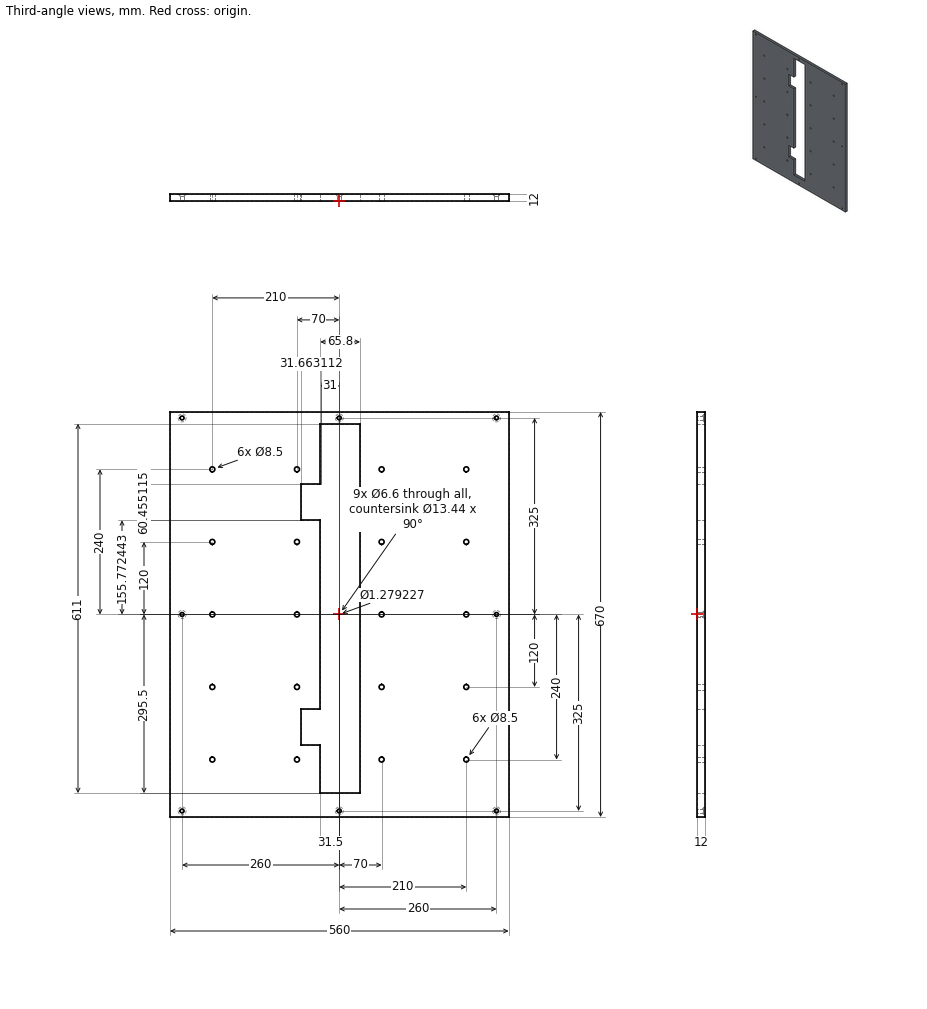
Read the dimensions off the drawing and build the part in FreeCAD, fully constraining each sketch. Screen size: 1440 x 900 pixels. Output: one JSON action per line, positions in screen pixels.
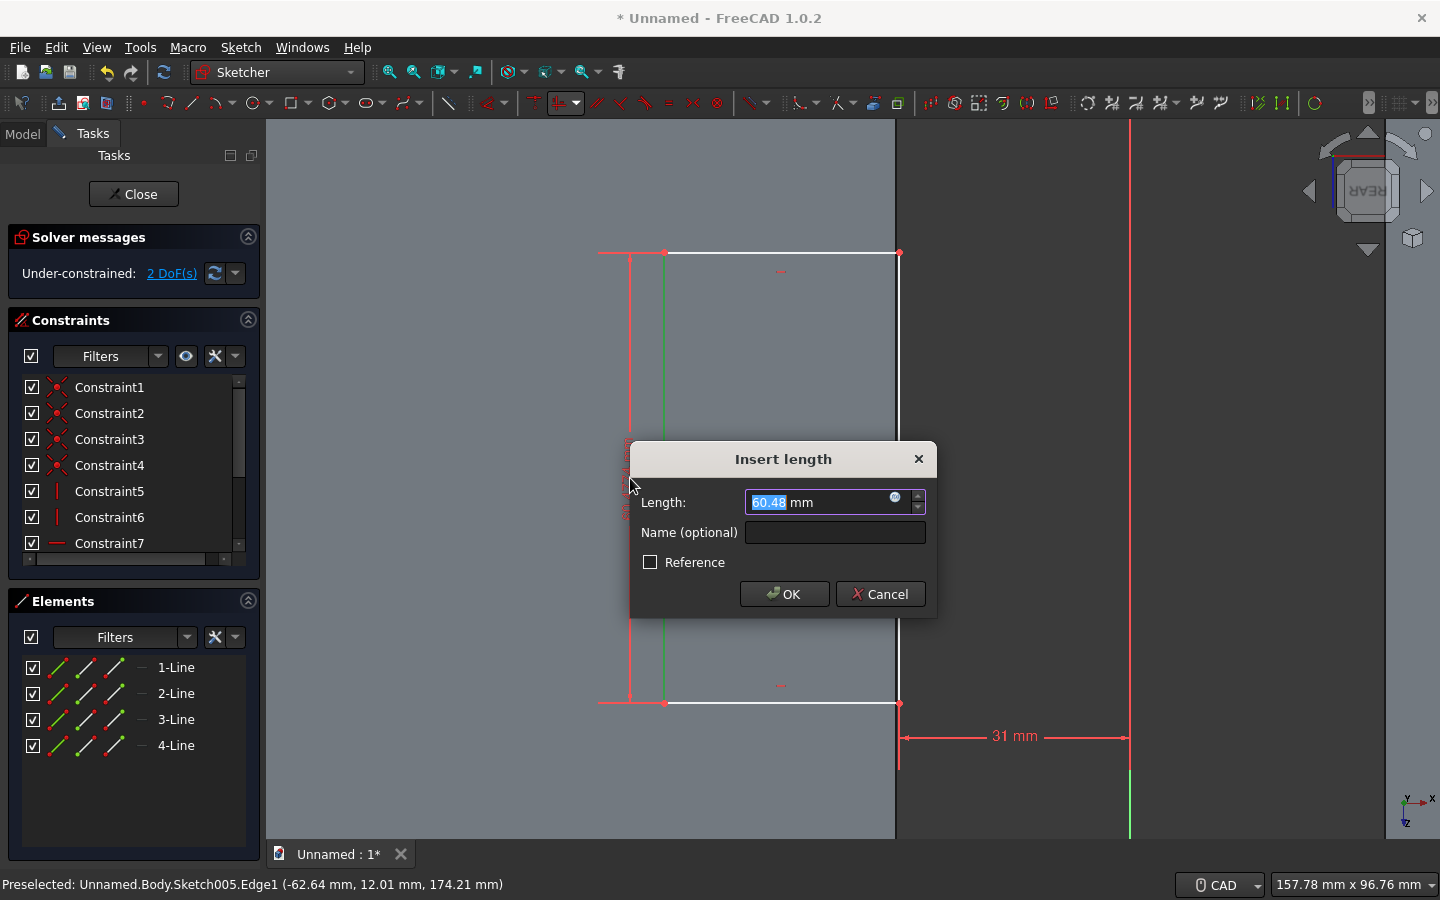
{"action": "type", "text": "60.455115"}
{"action": "key", "text": "Return"}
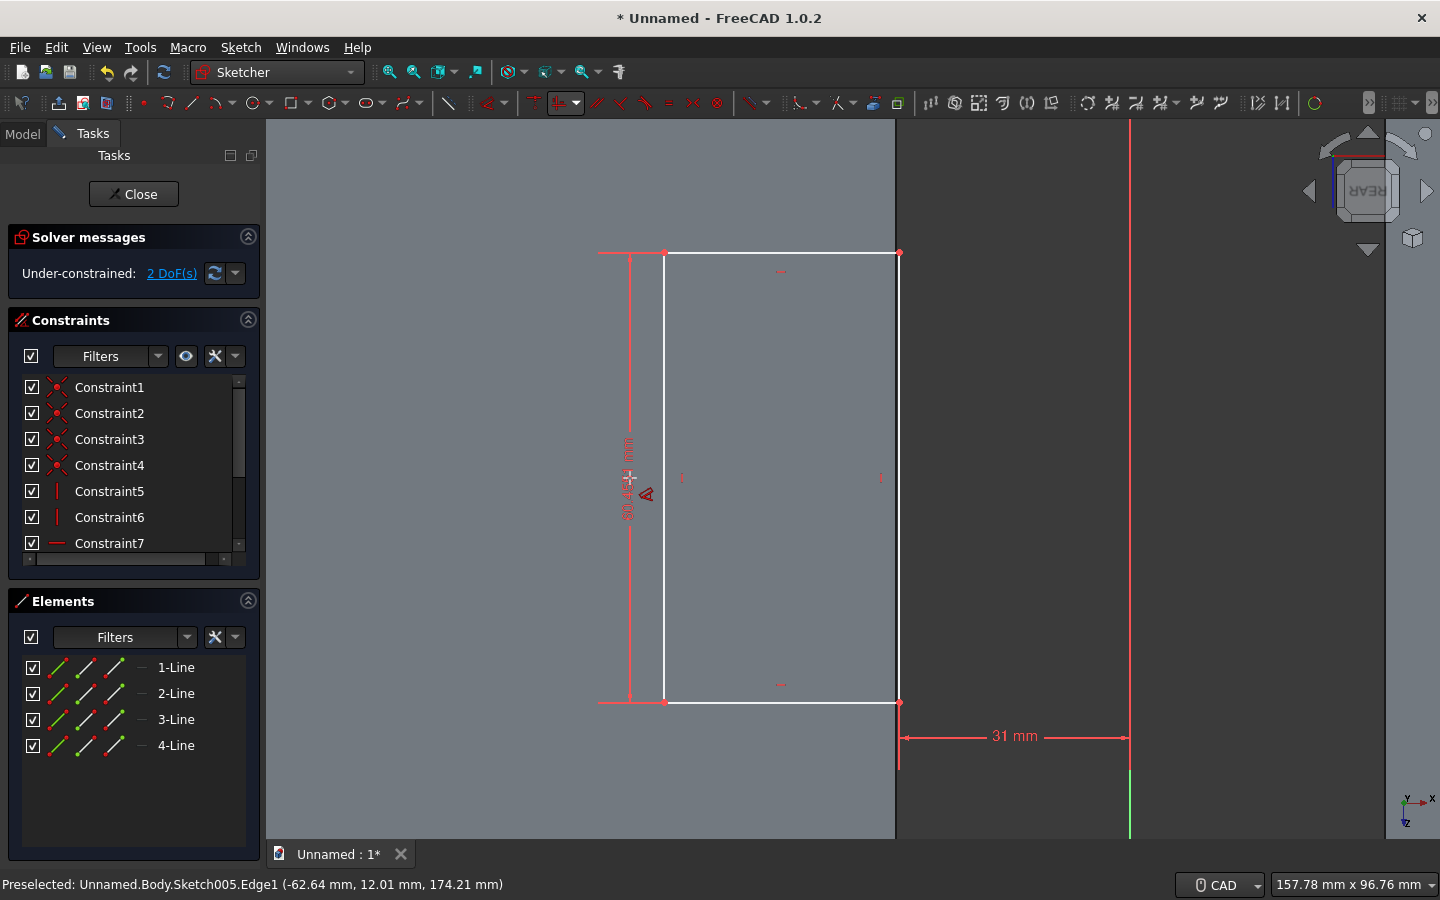
{"action": "left_click", "coordinate": [735, 703]}
{"action": "left_click", "coordinate": [782, 737]}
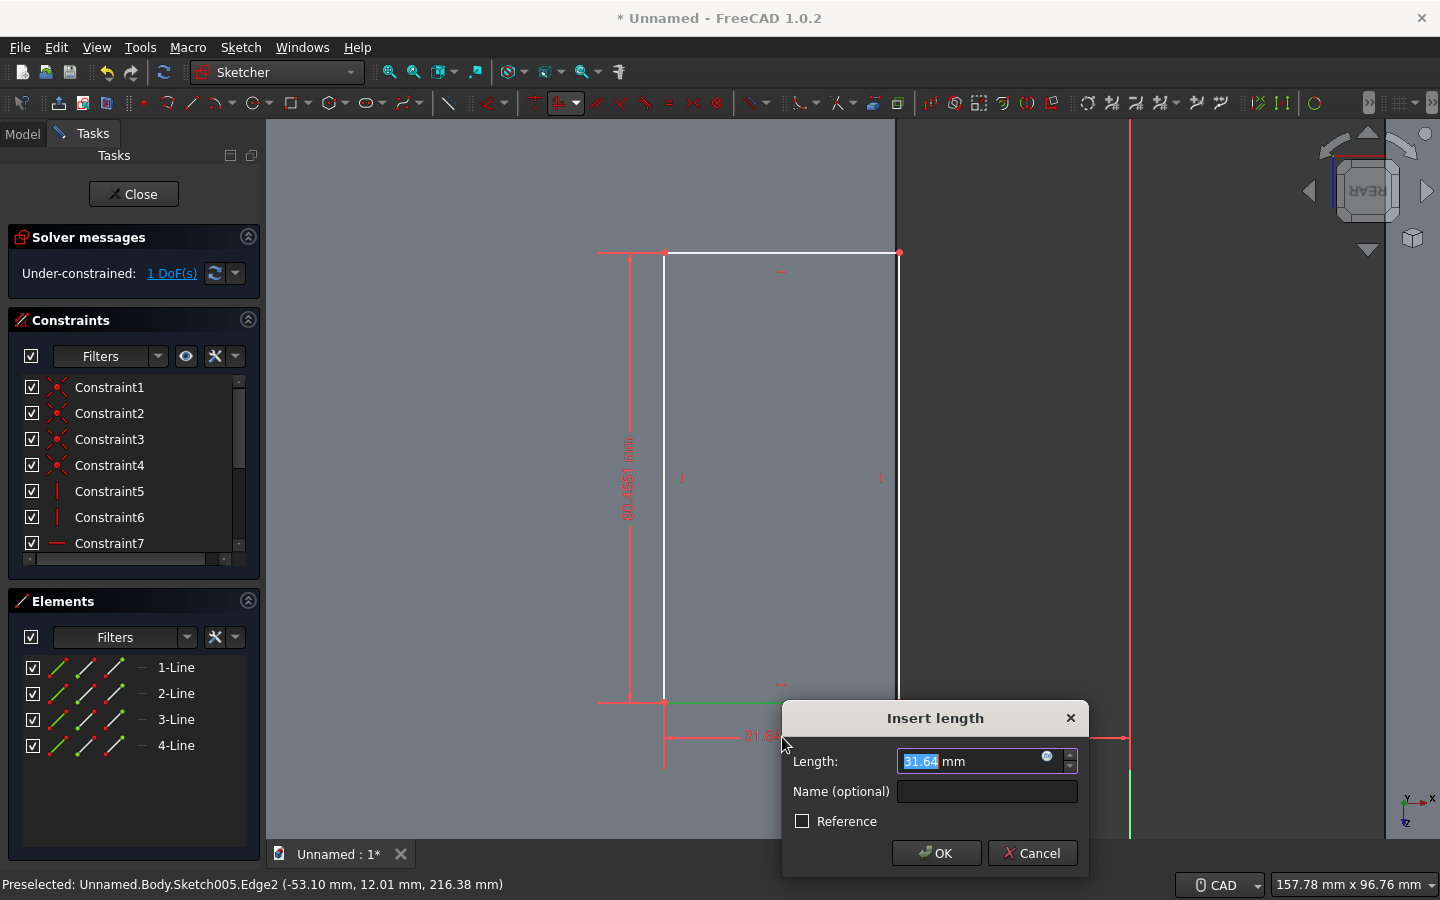
{"action": "type", "text": "31.663112"}
{"action": "key", "text": "Return"}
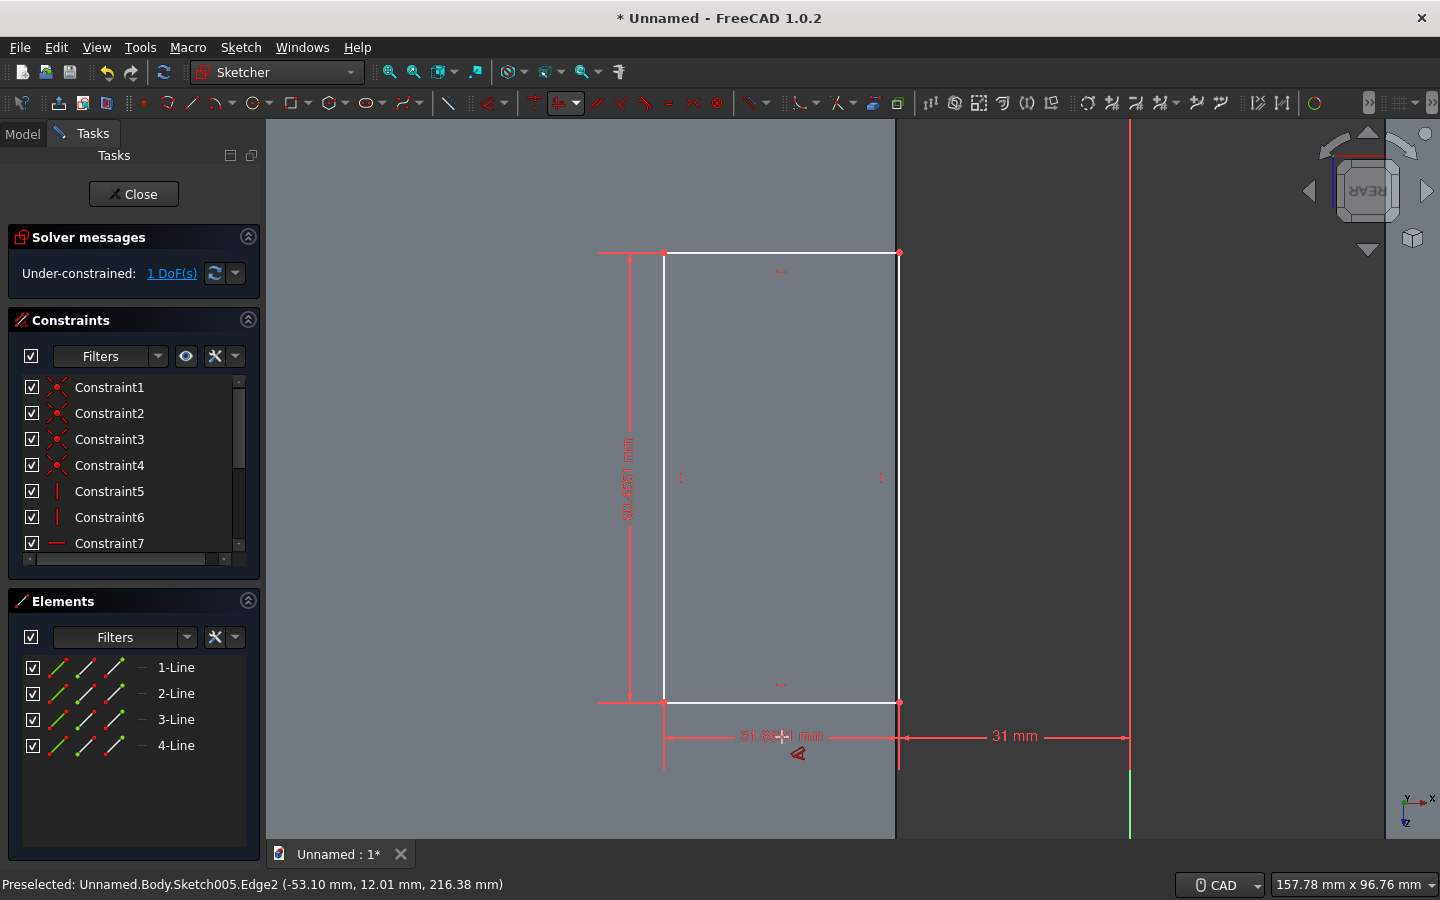
{"action": "left_click", "coordinate": [664, 253]}
{"action": "left_click", "coordinate": [1164, 200]}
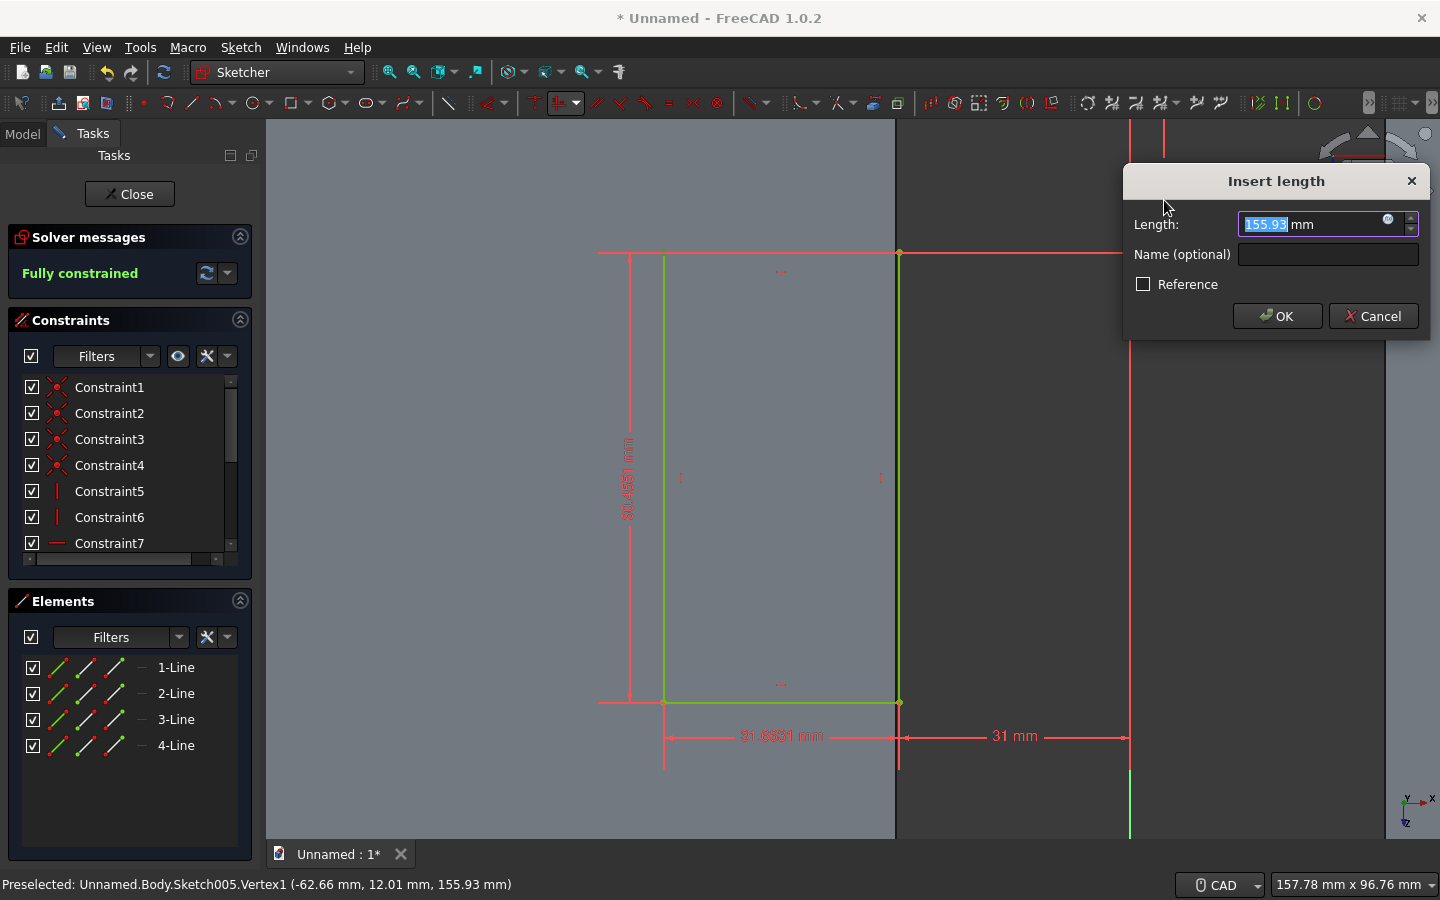
{"action": "type", "text": "155.772443"}
{"action": "key", "text": "Return"}
{"action": "key", "text": "Escape"}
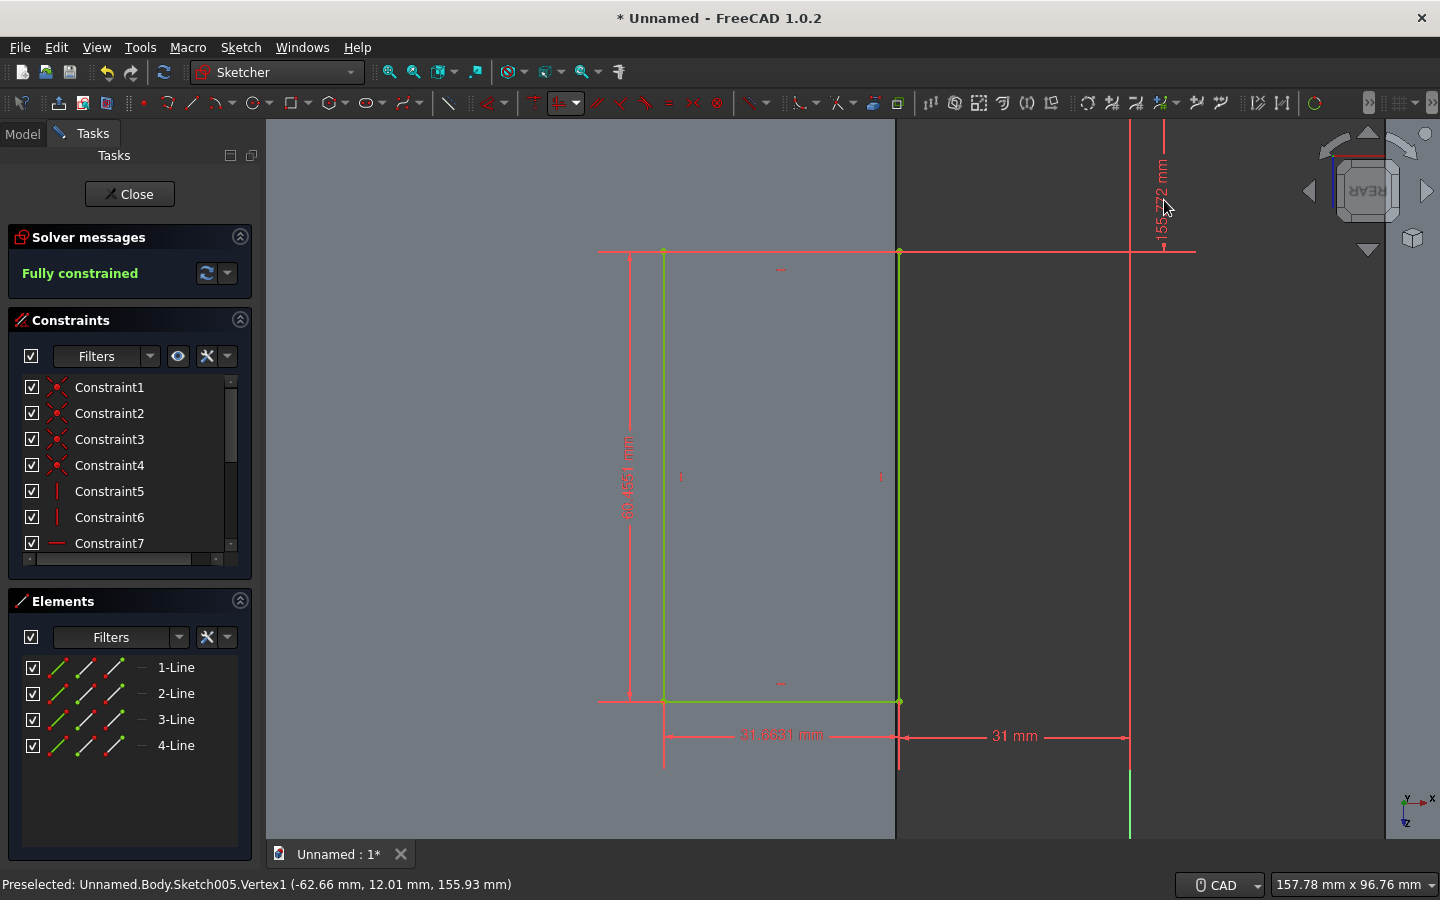
{"action": "left_click", "coordinate": [130, 194]}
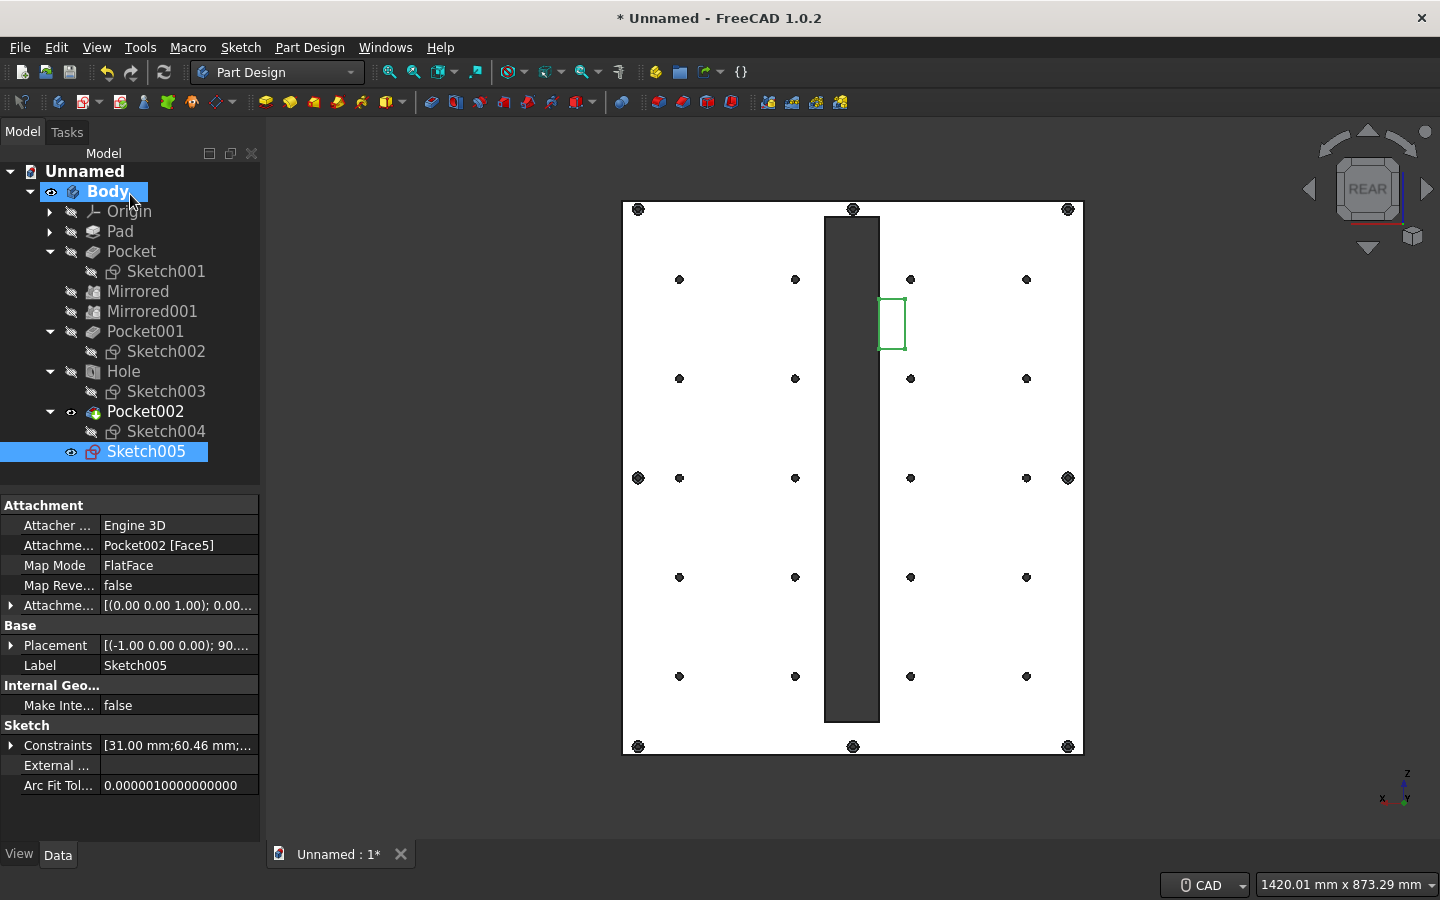
{"action": "left_click", "coordinate": [432, 102]}